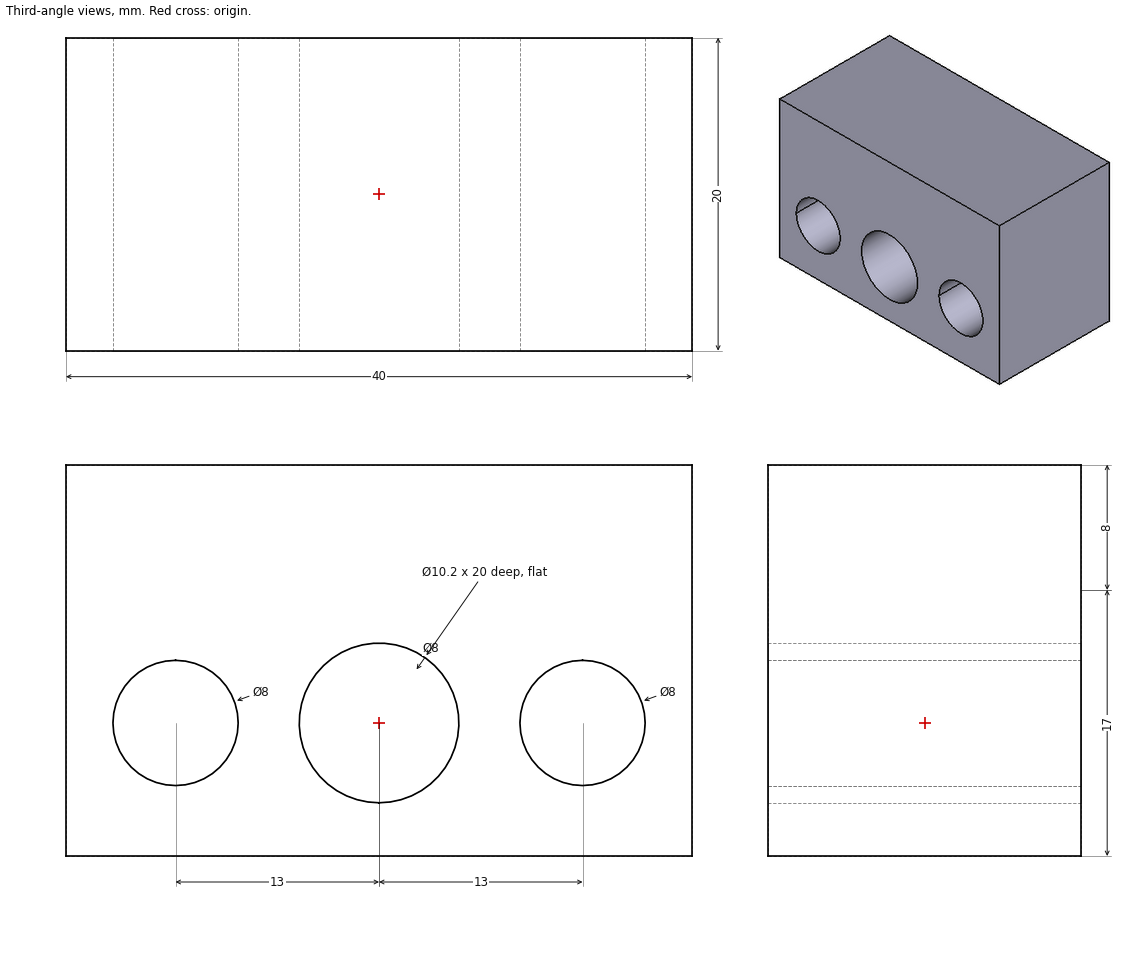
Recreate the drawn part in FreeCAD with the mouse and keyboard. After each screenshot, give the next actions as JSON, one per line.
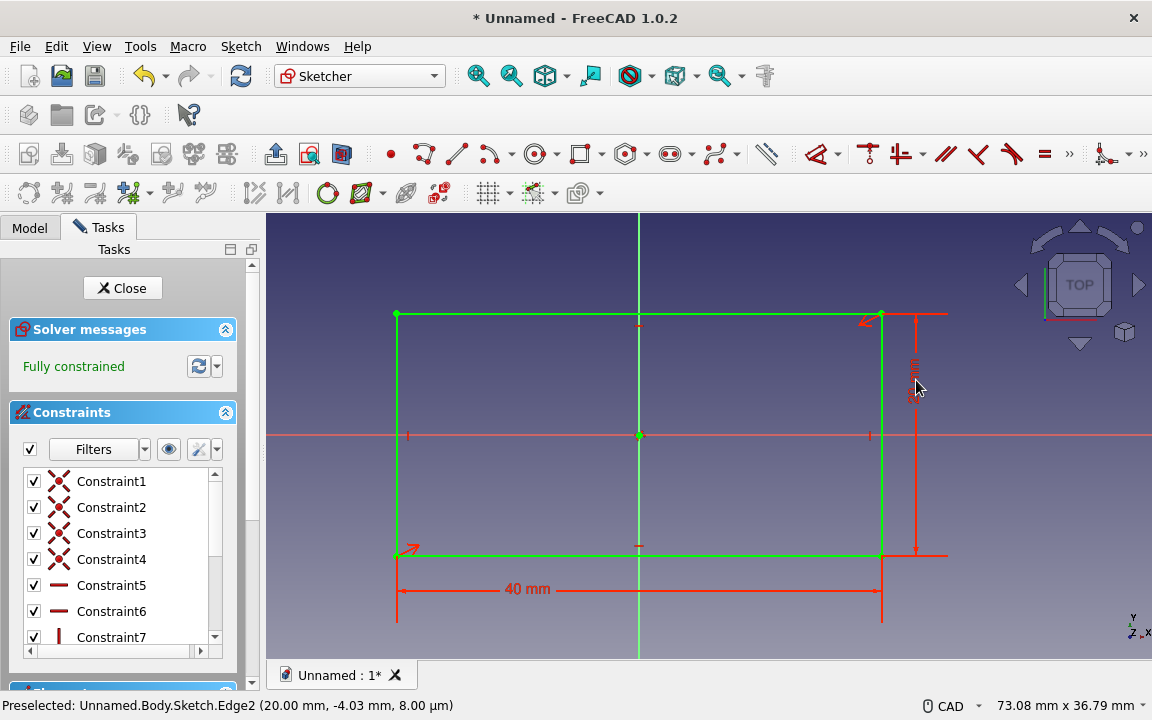
{"action": "left_click", "coordinate": [123, 288]}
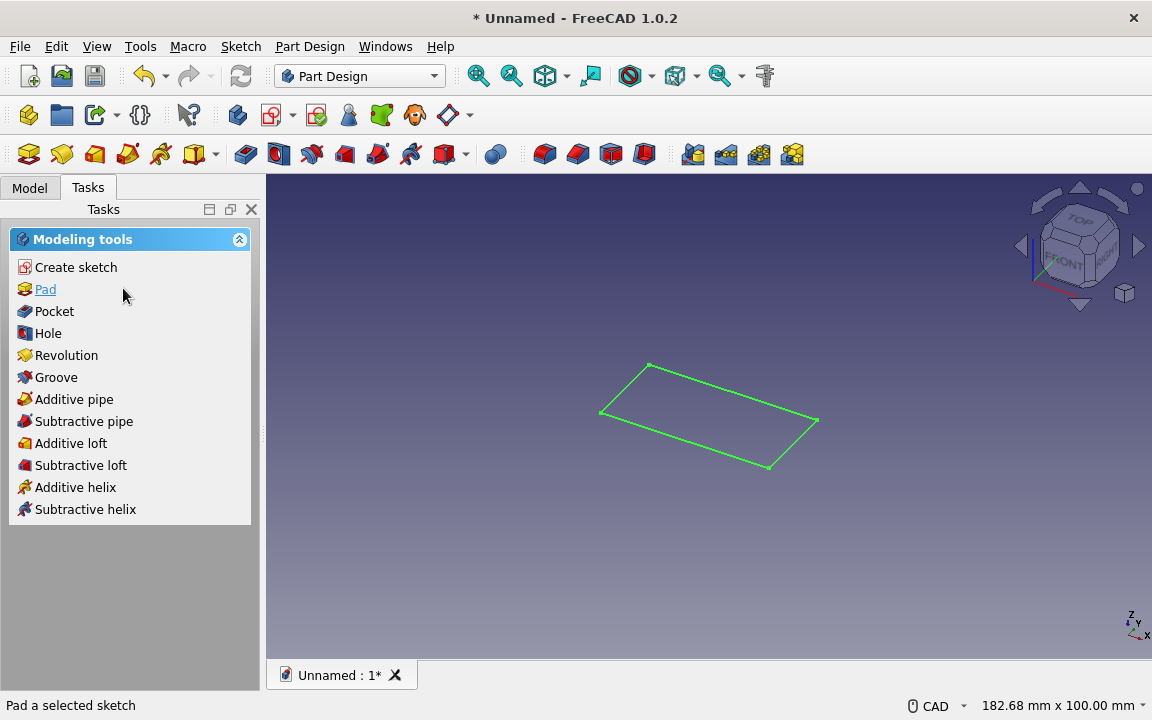
{"action": "left_click", "coordinate": [29, 154]}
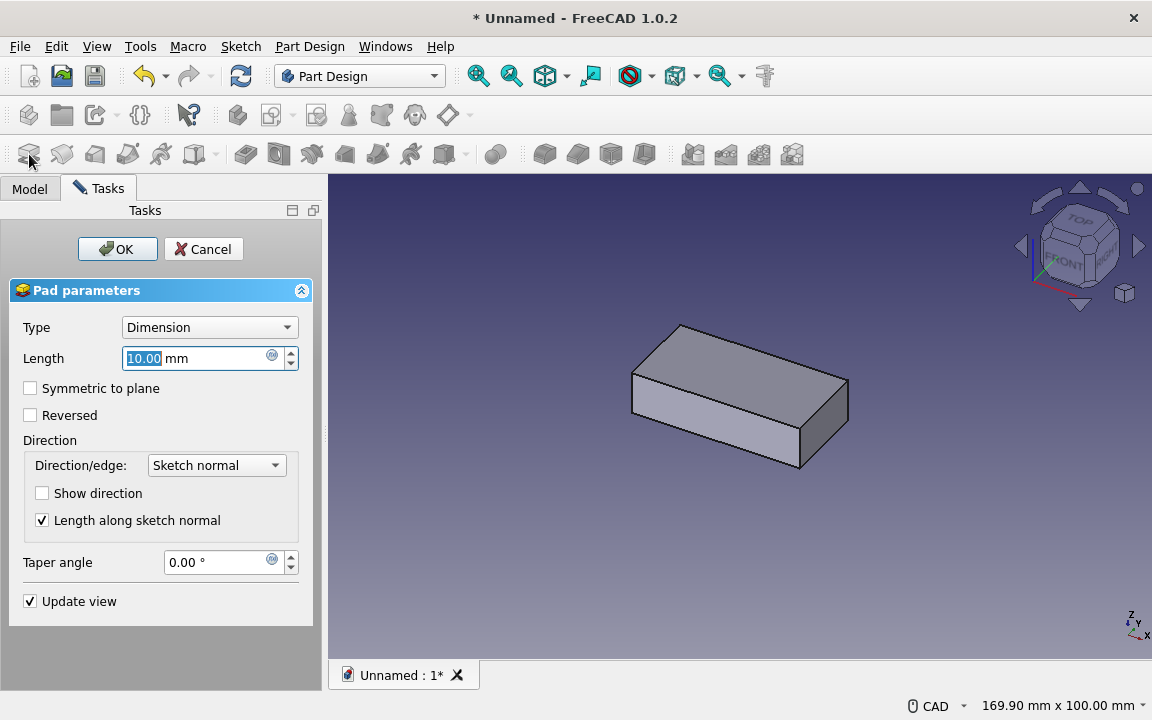
{"action": "type", "text": "17"}
{"action": "key", "text": "Tab"}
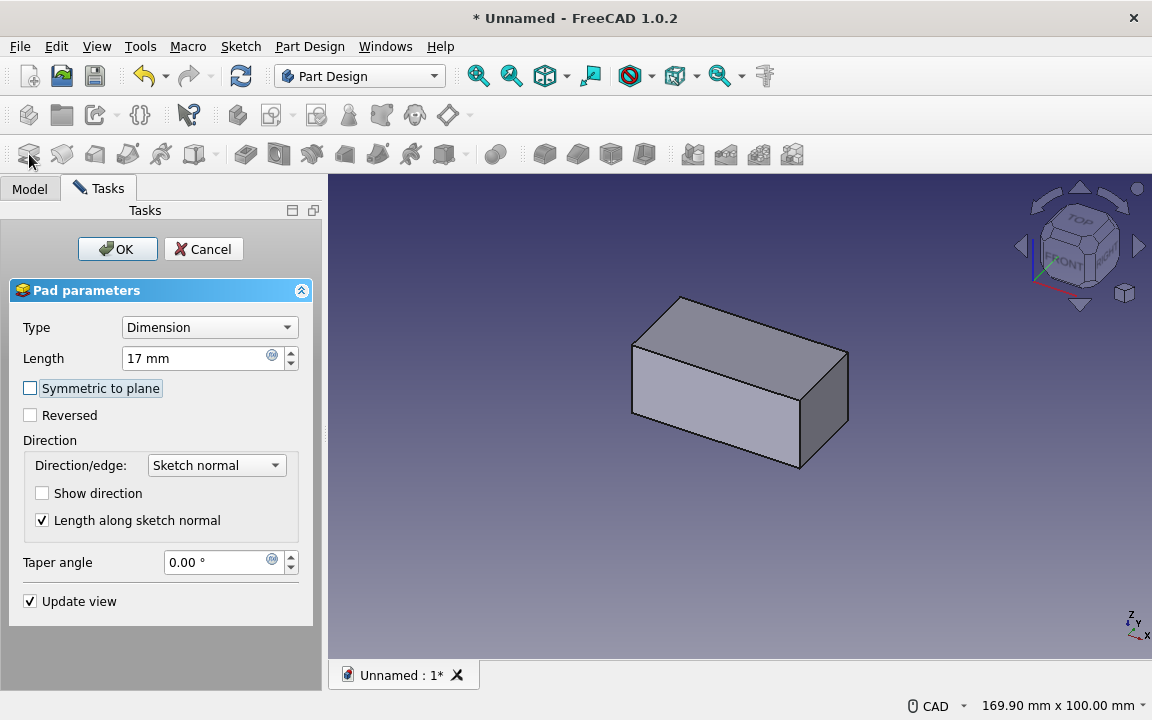
{"action": "left_click", "coordinate": [31, 388]}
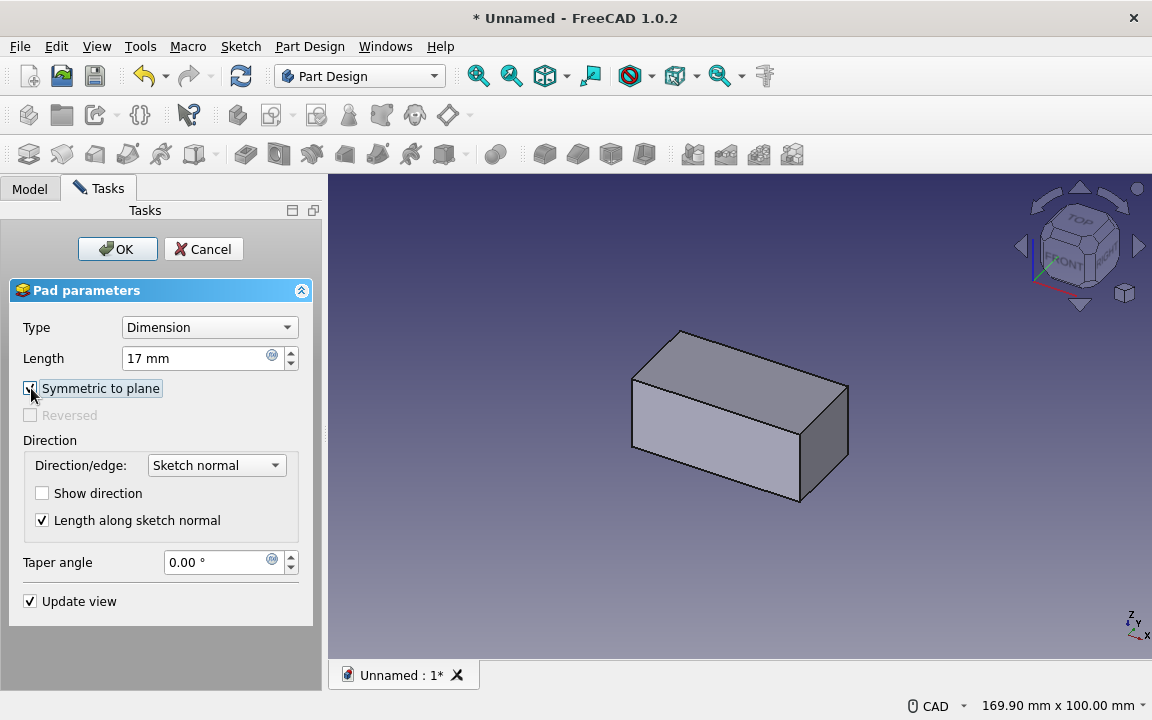
{"action": "left_click", "coordinate": [118, 249]}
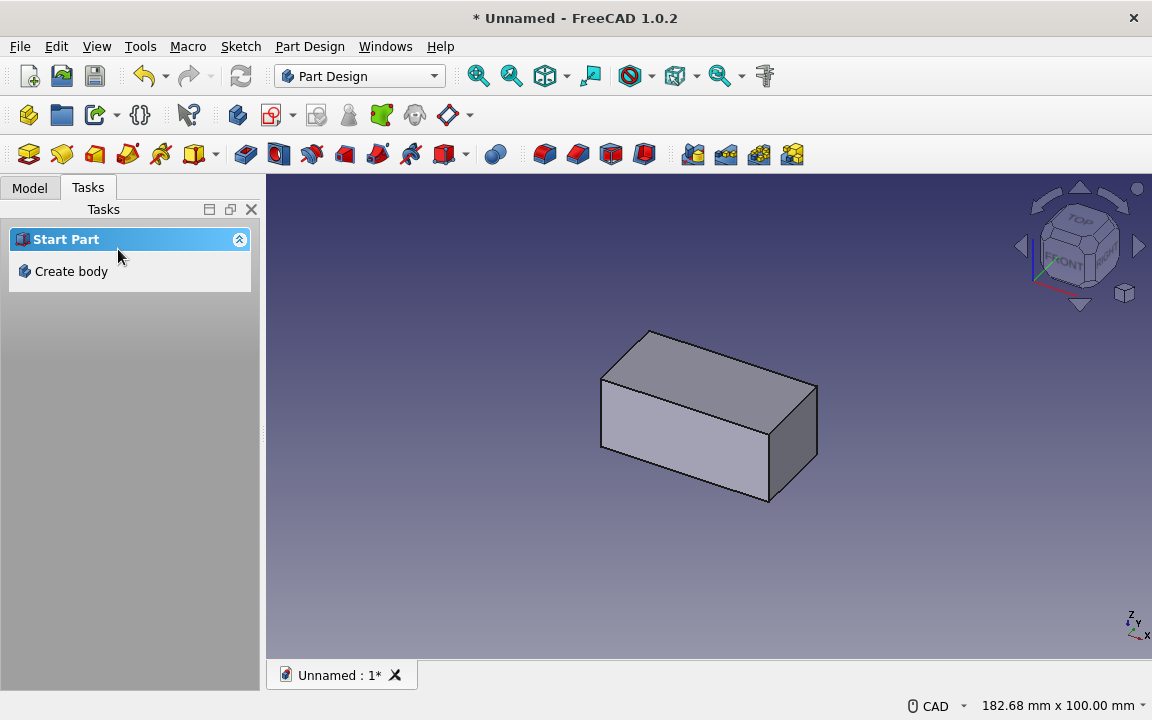
{"action": "left_click", "coordinate": [479, 76]}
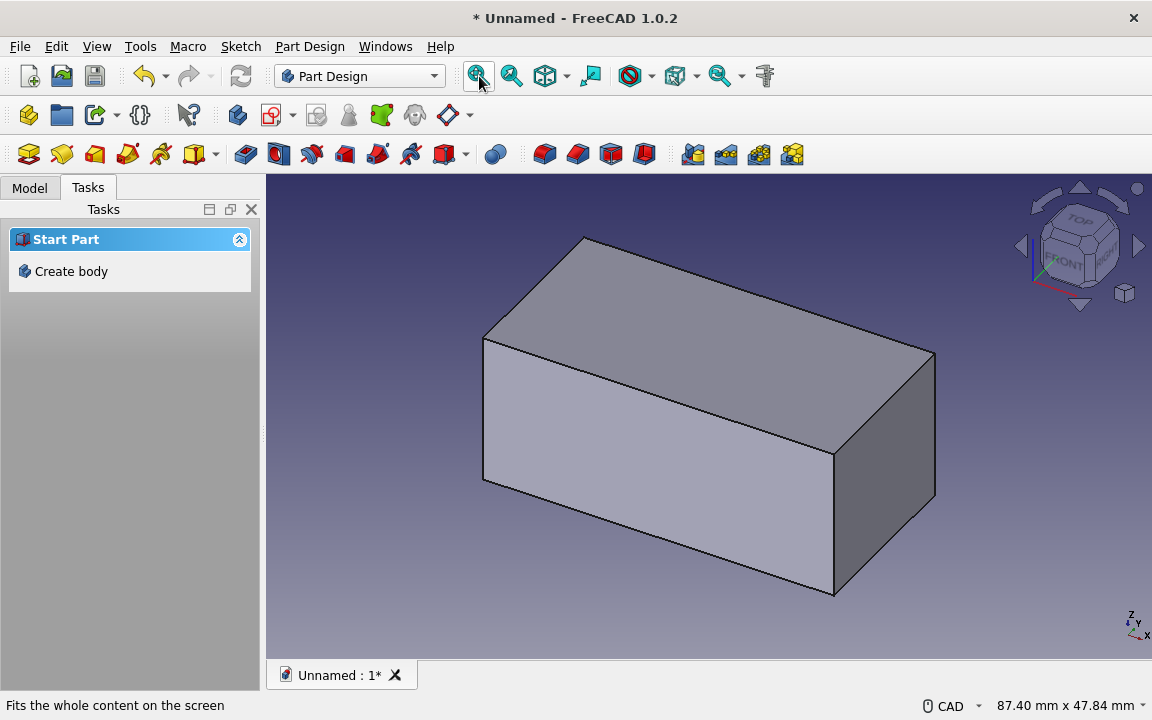
{"action": "key", "text": "4"}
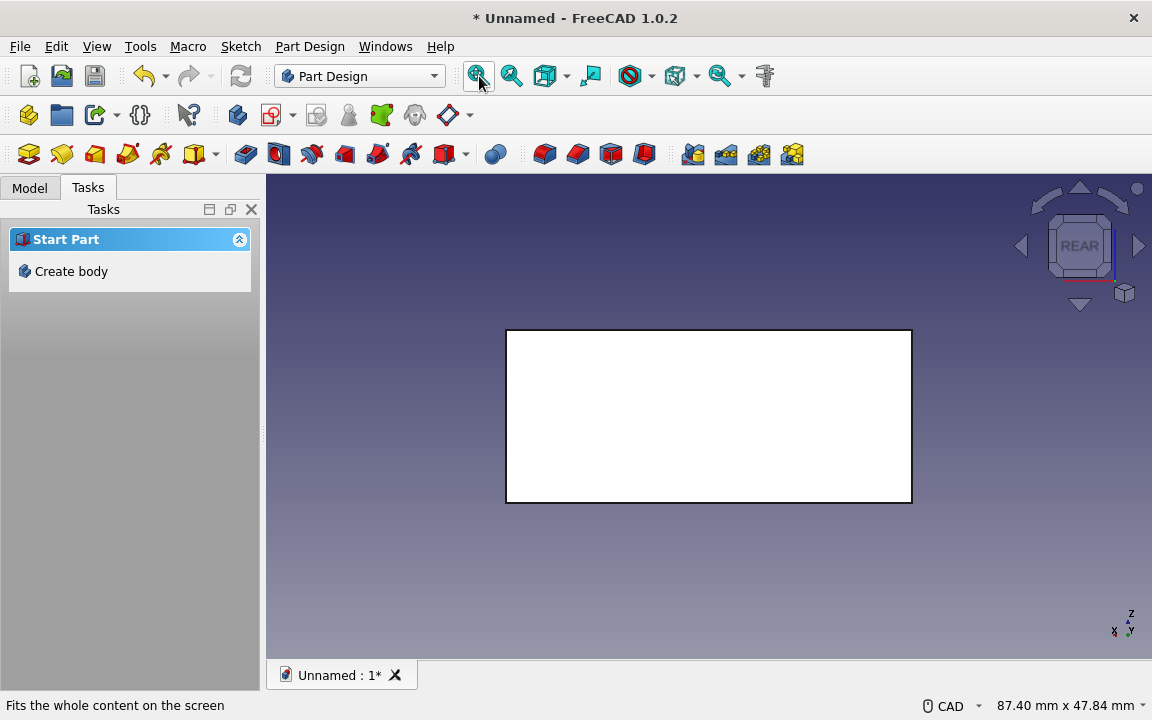
{"action": "left_click", "coordinate": [593, 415]}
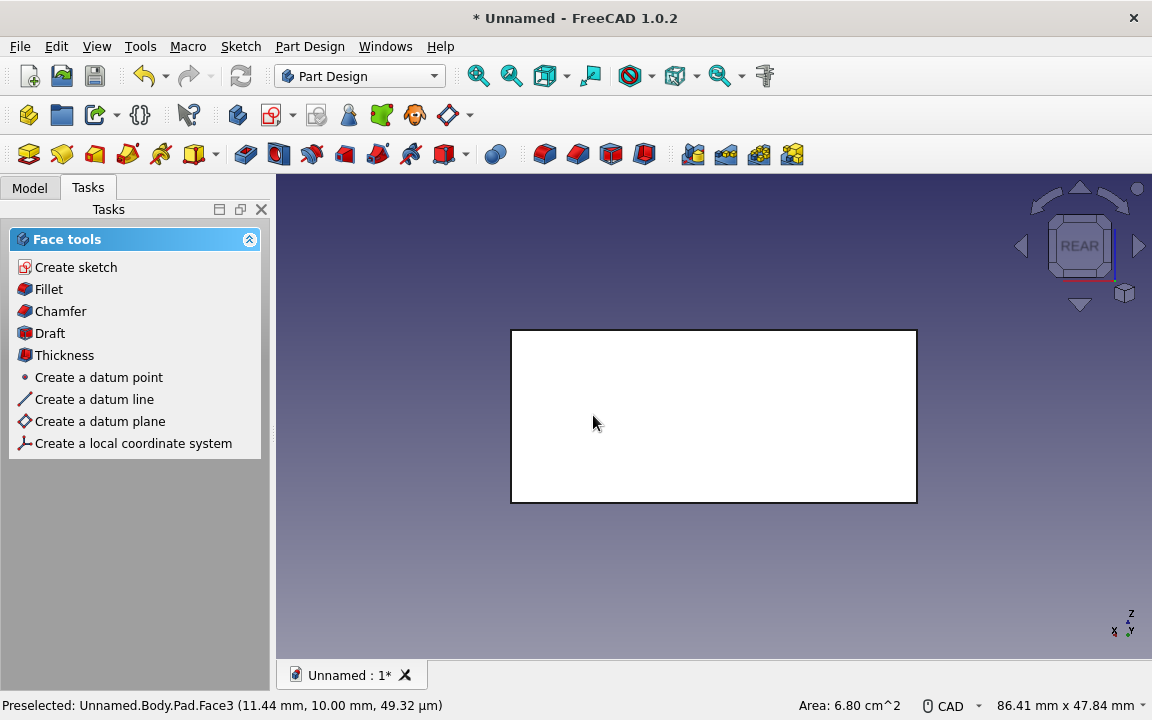
{"action": "left_click", "coordinate": [270, 116]}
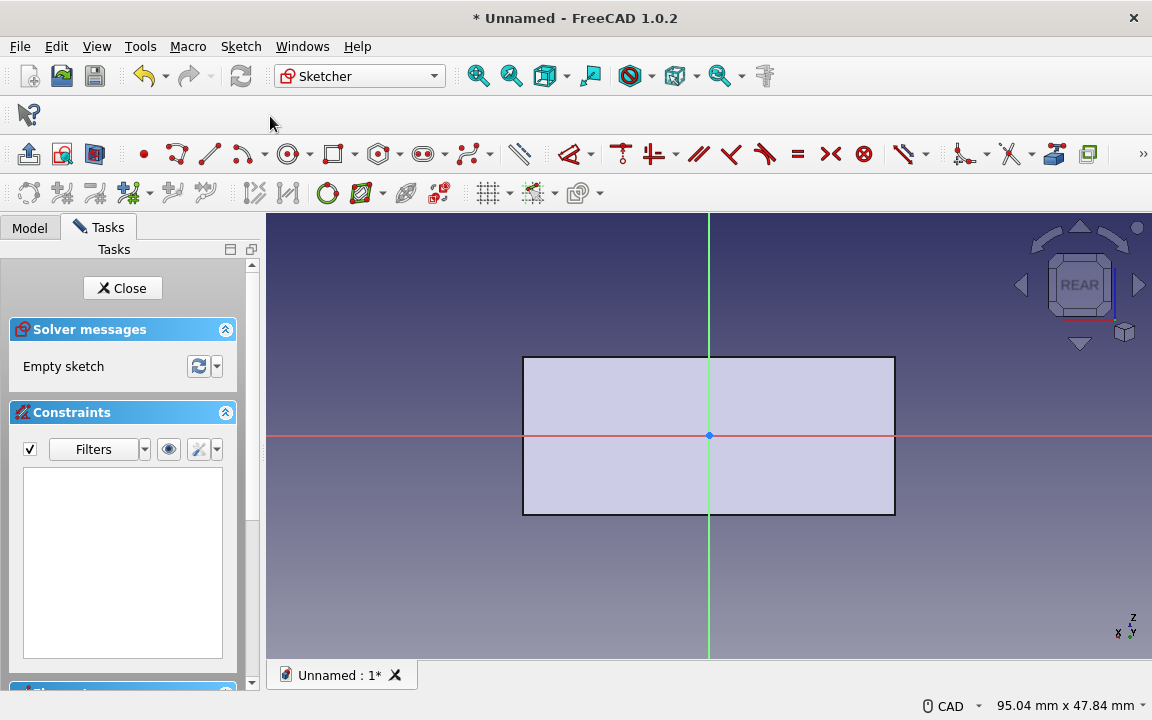
{"action": "scroll", "coordinate": [852, 436], "scroll_direction": "up", "scroll_amount": 6}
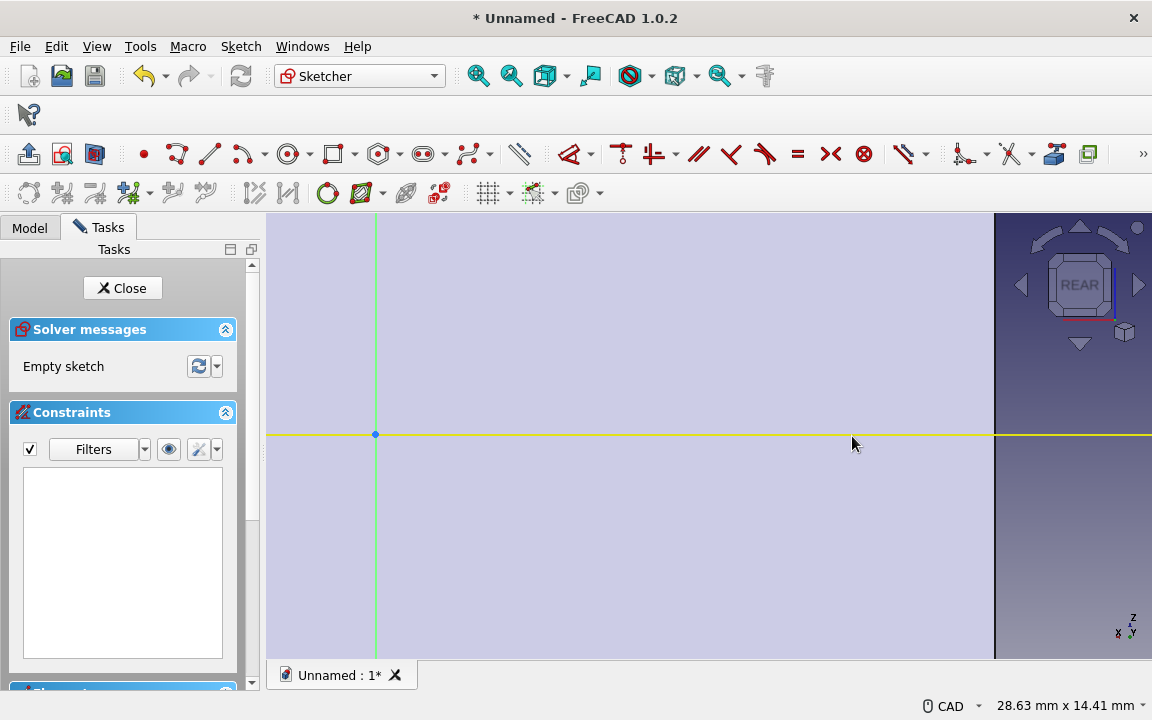
{"action": "left_click", "coordinate": [288, 154]}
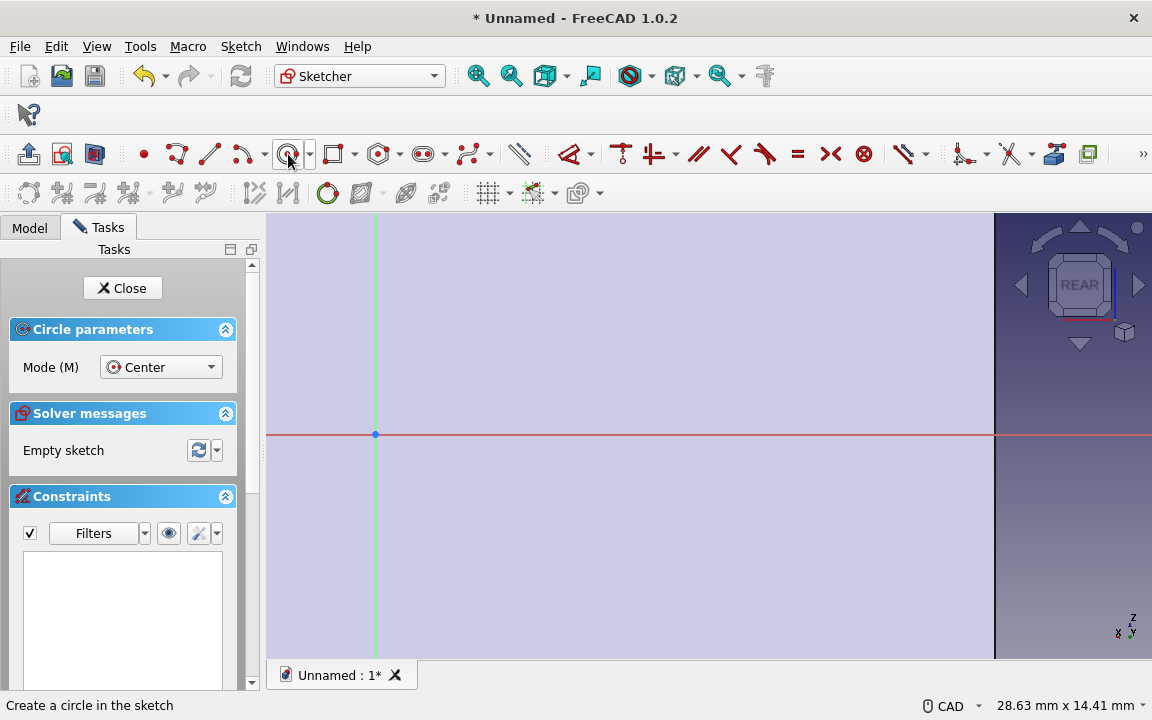
{"action": "left_click", "coordinate": [778, 435]}
{"action": "left_click", "coordinate": [866, 347]}
{"action": "key", "text": "Escape"}